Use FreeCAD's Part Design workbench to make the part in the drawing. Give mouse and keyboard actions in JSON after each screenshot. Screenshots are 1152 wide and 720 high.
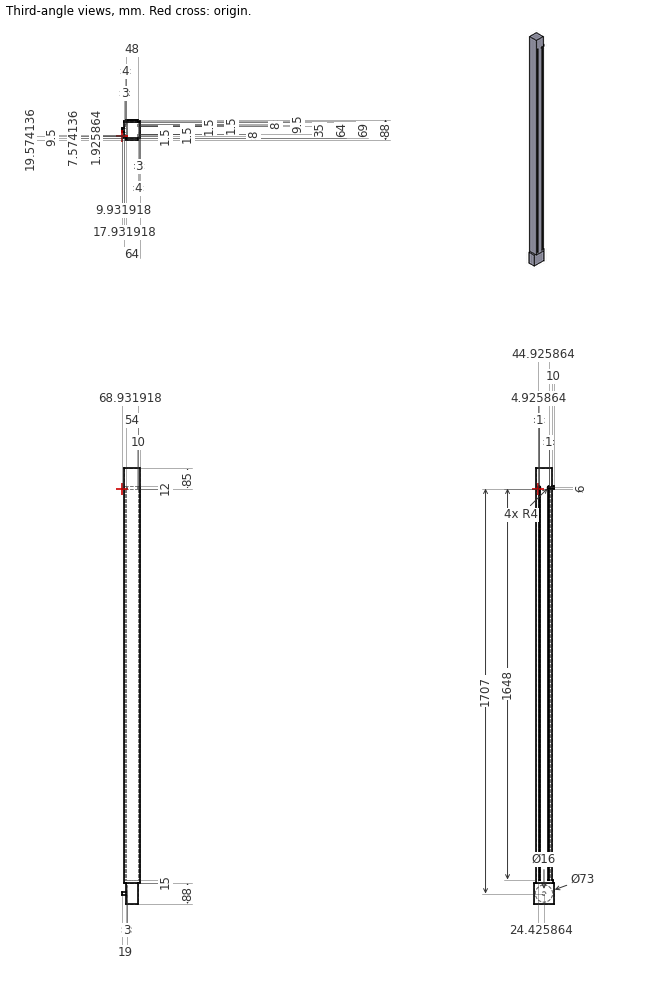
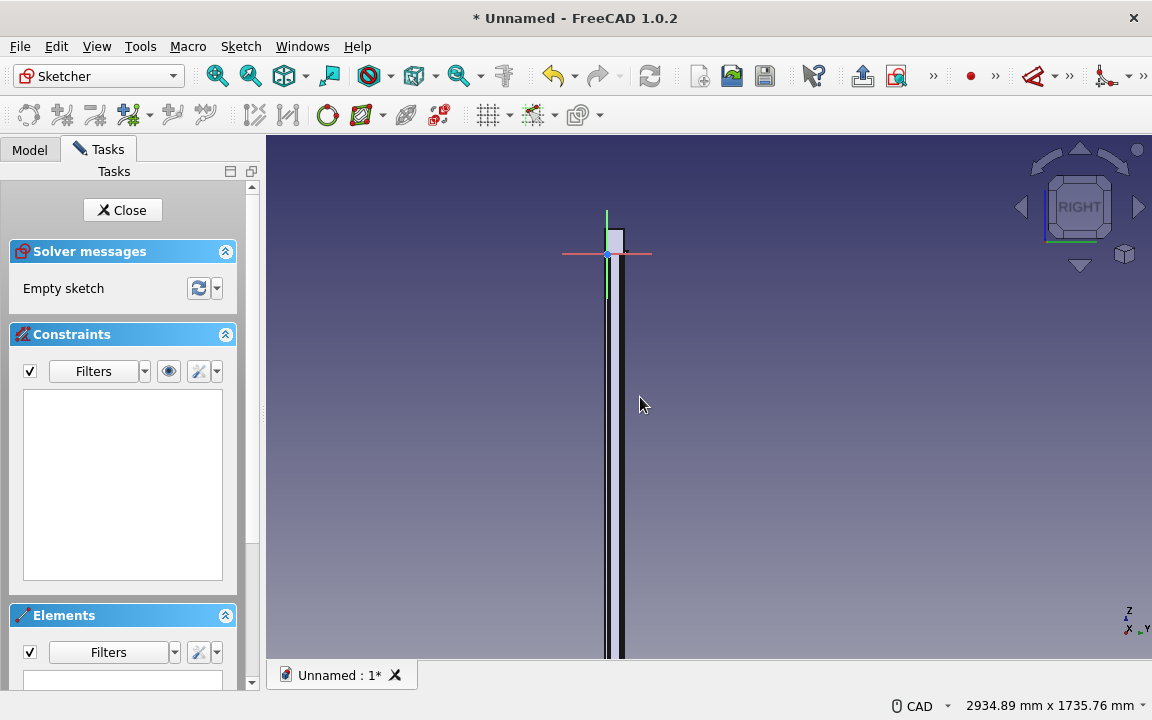
{"action": "scroll", "coordinate": [613, 245], "scroll_direction": "up", "scroll_amount": 15}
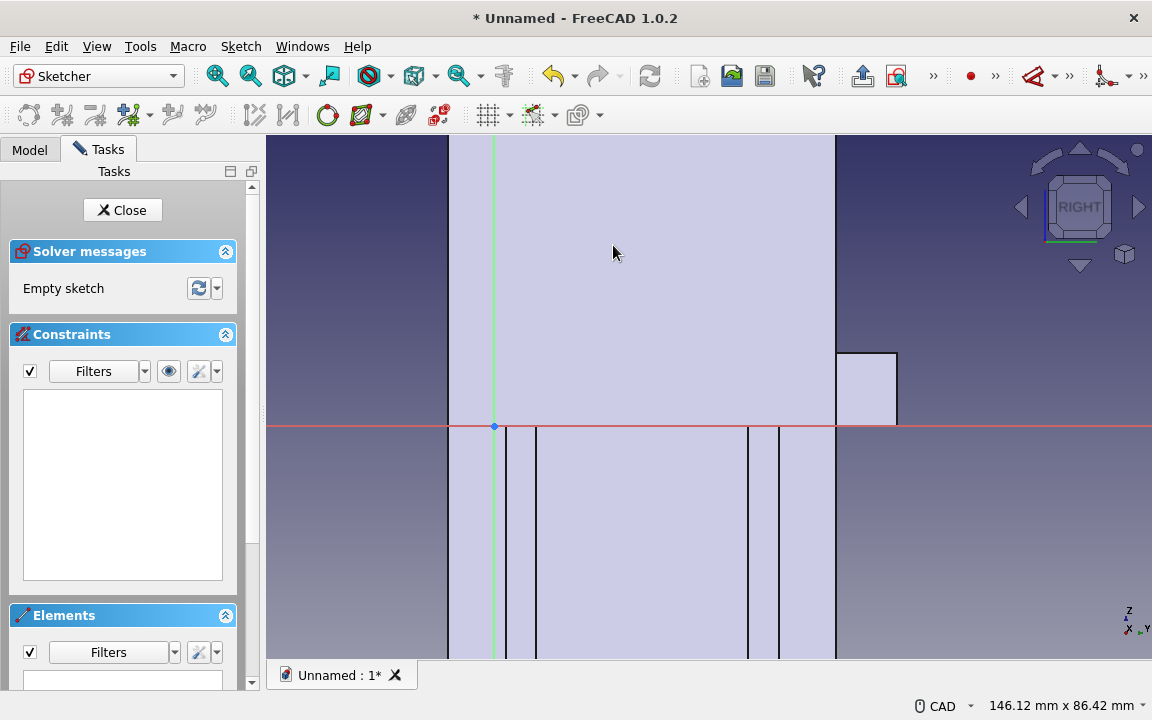
{"action": "scroll", "coordinate": [645, 393], "scroll_direction": "up", "scroll_amount": 2}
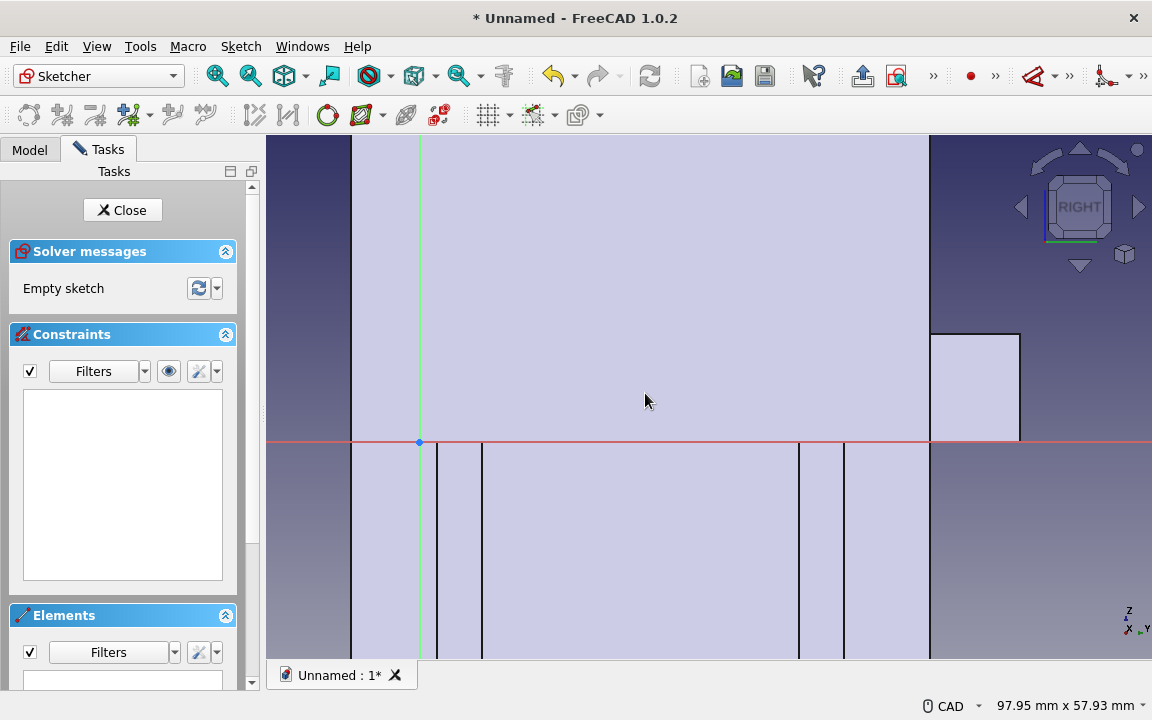
{"action": "key", "text": "g l"}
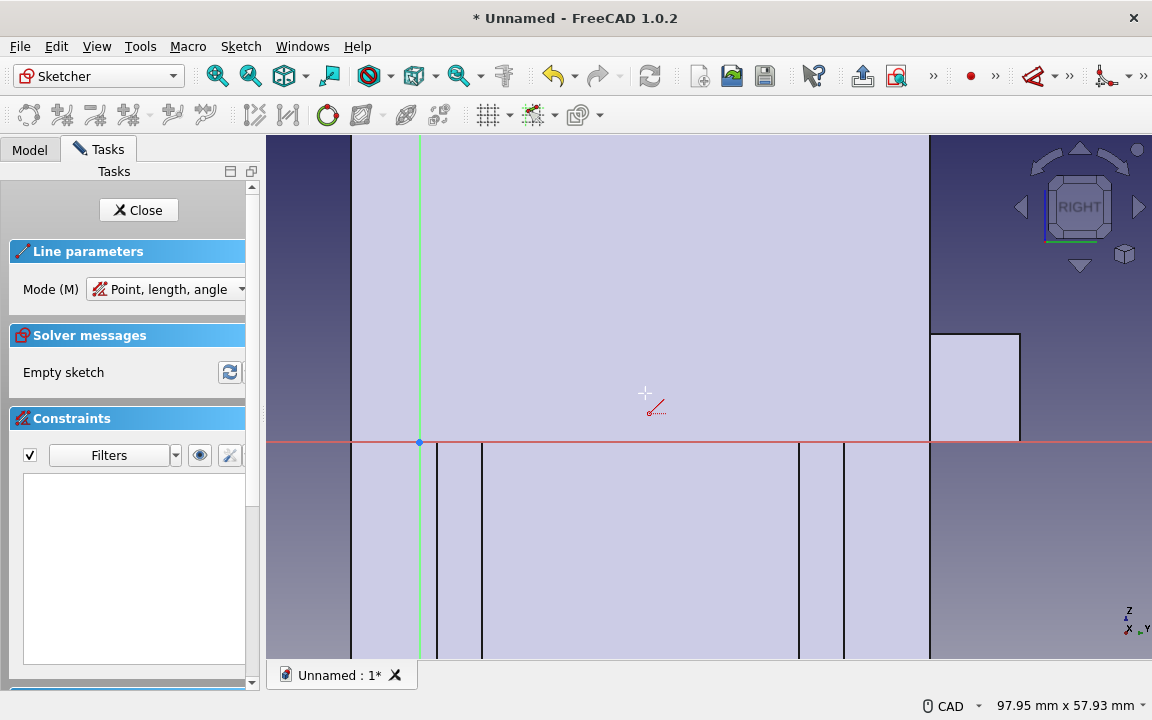
{"action": "left_click", "coordinate": [826, 352]}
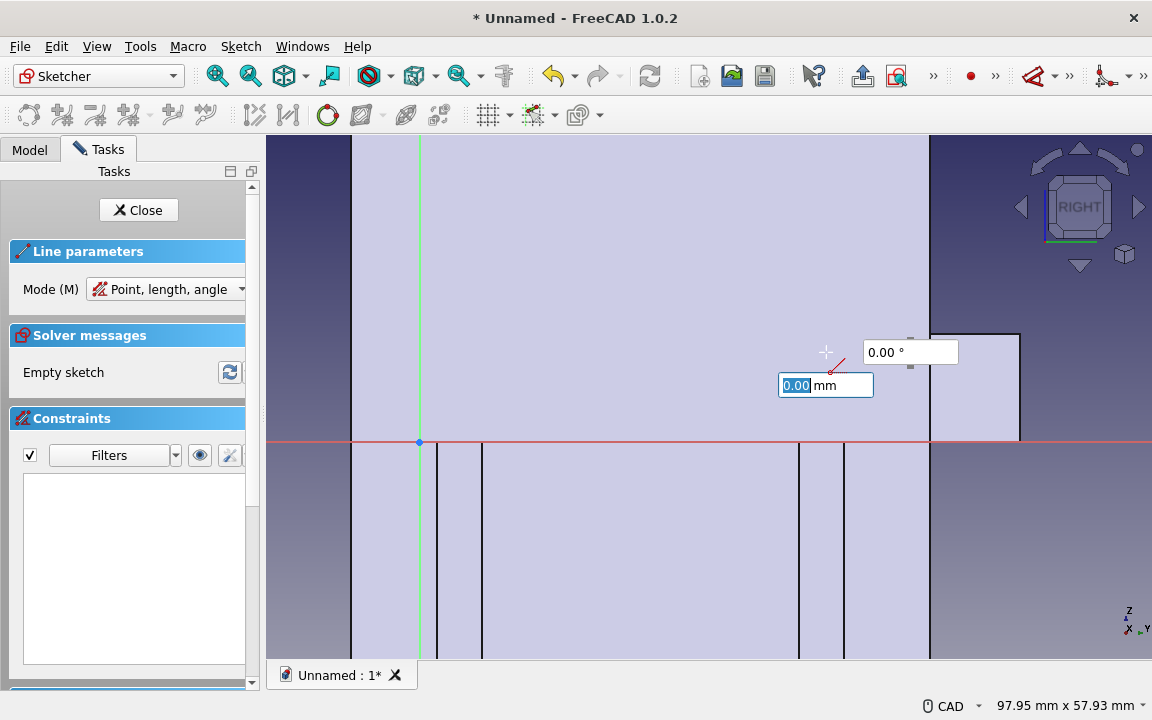
{"action": "scroll", "coordinate": [817, 352], "scroll_direction": "up", "scroll_amount": 3}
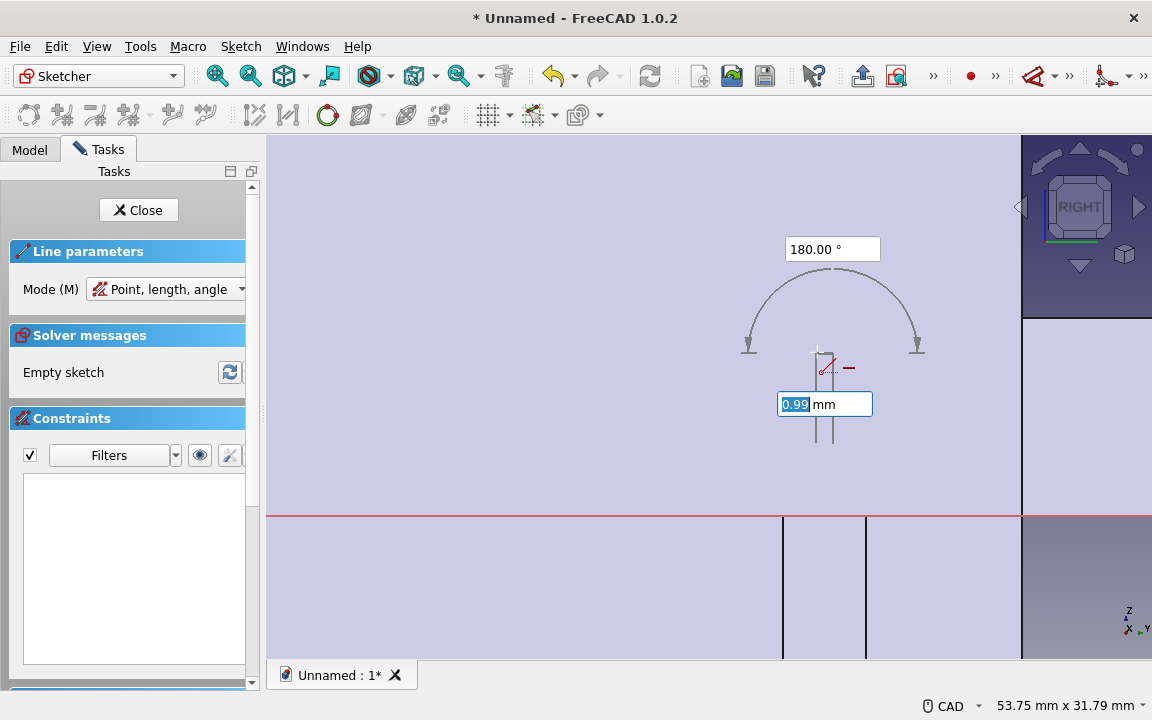
{"action": "left_click", "coordinate": [816, 352]}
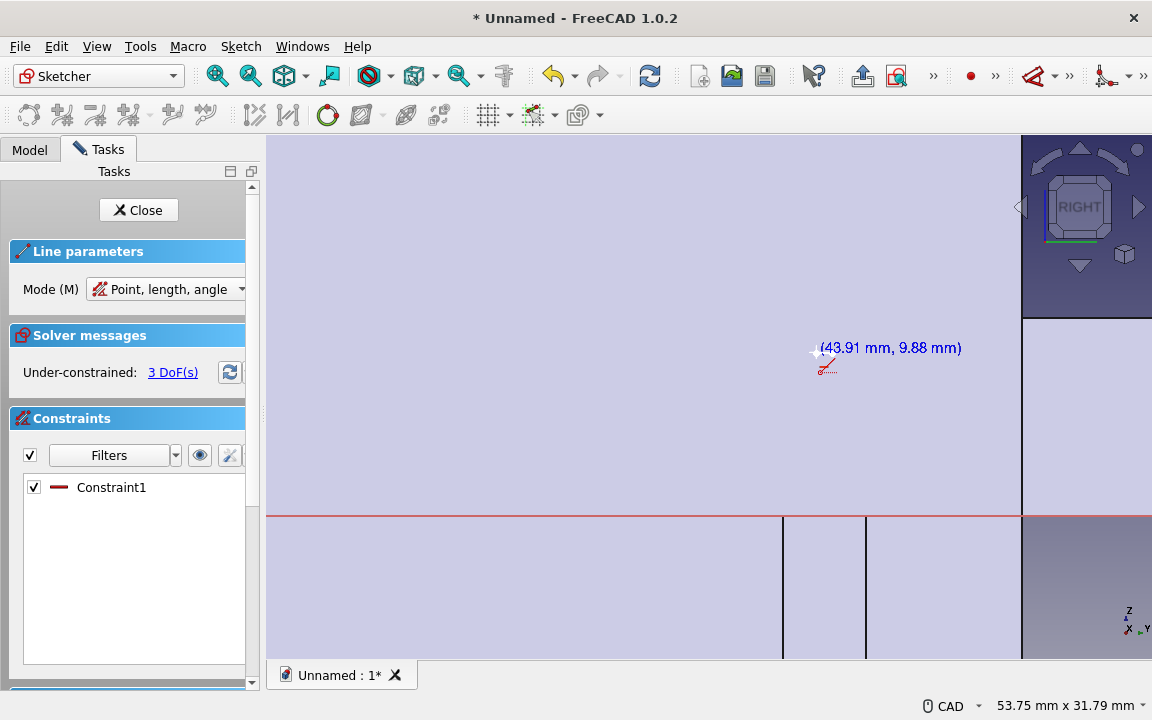
{"action": "key", "text": "g m"}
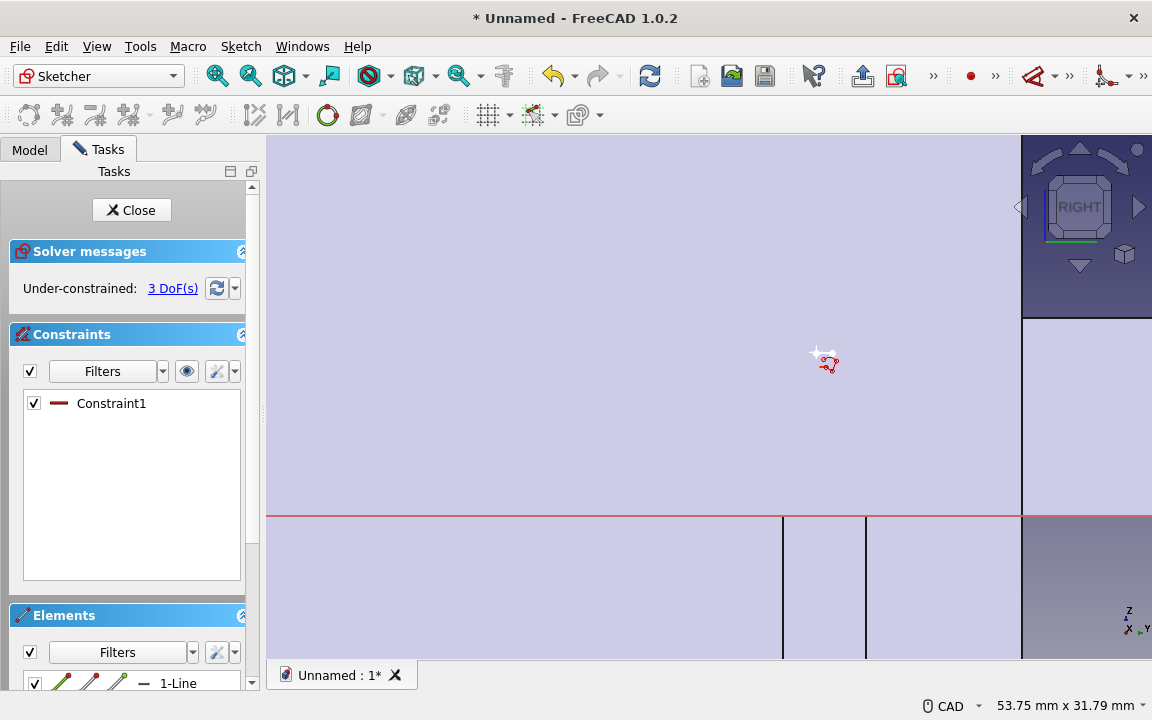
{"action": "left_click", "coordinate": [750, 417]}
{"action": "left_click", "coordinate": [750, 516]}
{"action": "left_click", "coordinate": [899, 507]}
{"action": "left_click", "coordinate": [899, 417]}
{"action": "right_click", "coordinate": [899, 417]}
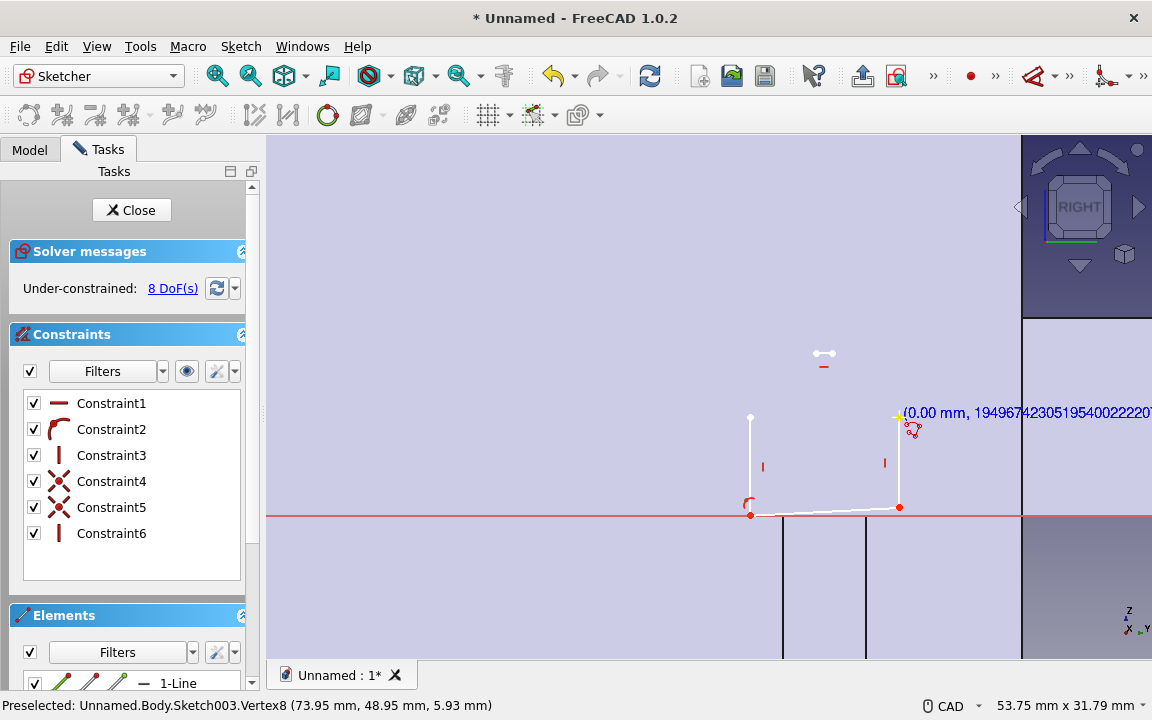
{"action": "key", "text": "g 3 a"}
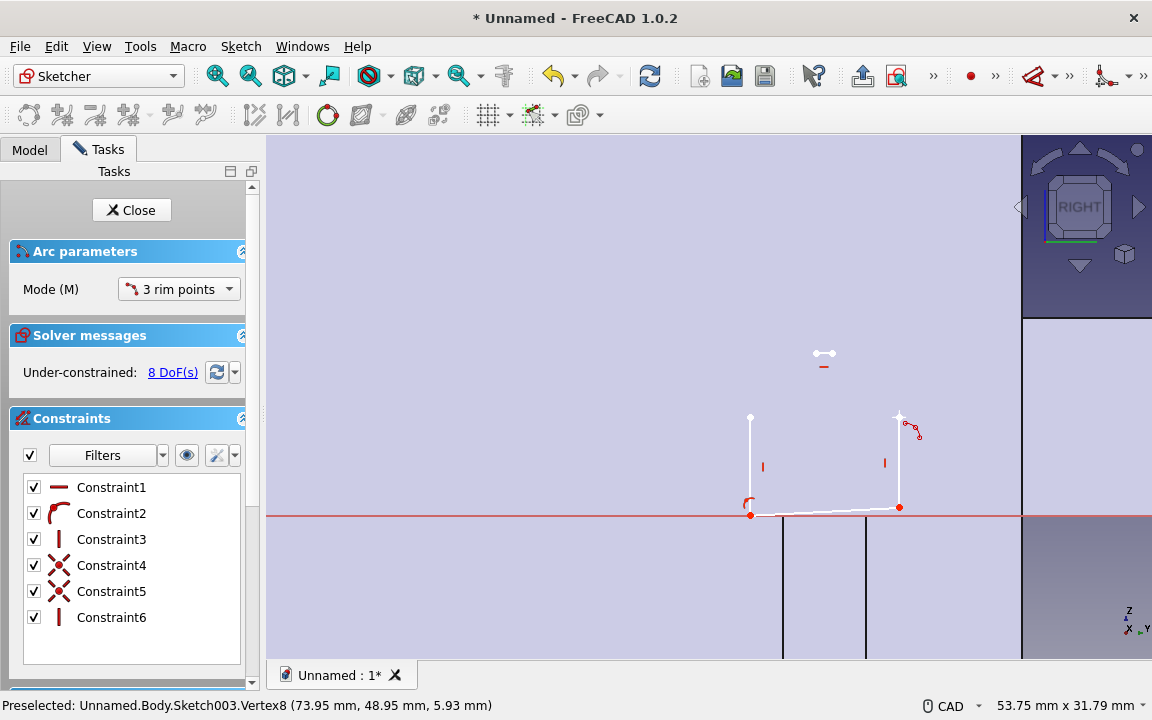
{"action": "scroll", "coordinate": [816, 351], "scroll_direction": "up", "scroll_amount": 4}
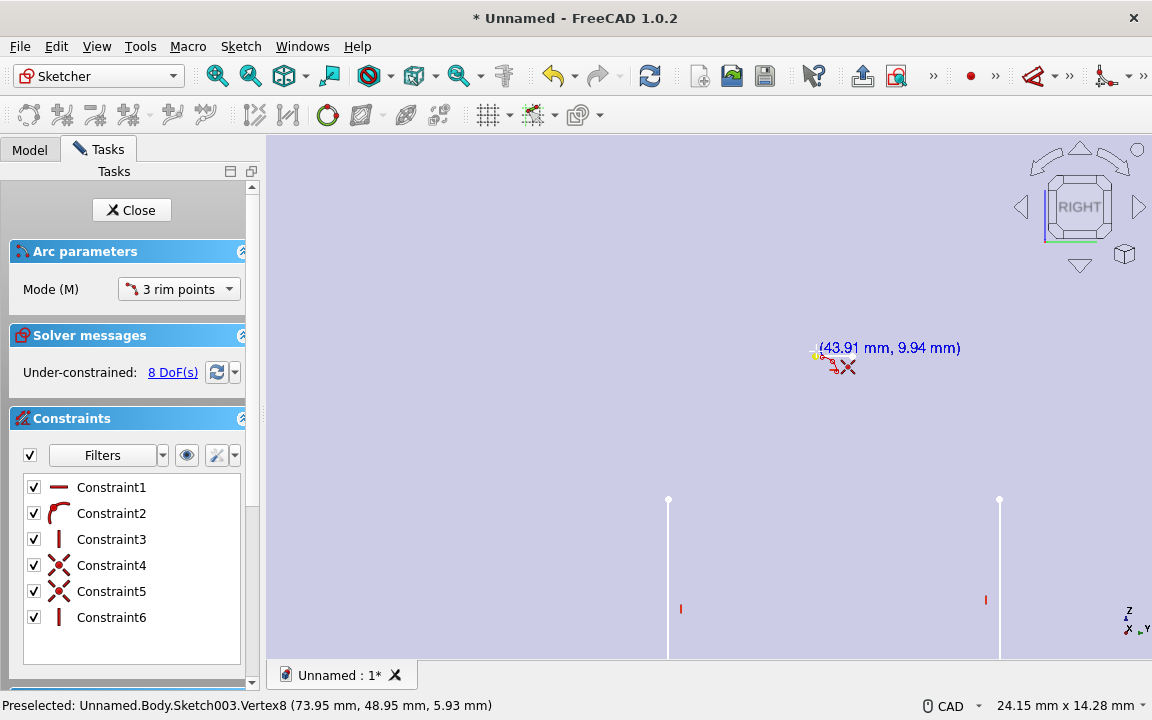
{"action": "left_click", "coordinate": [815, 356]}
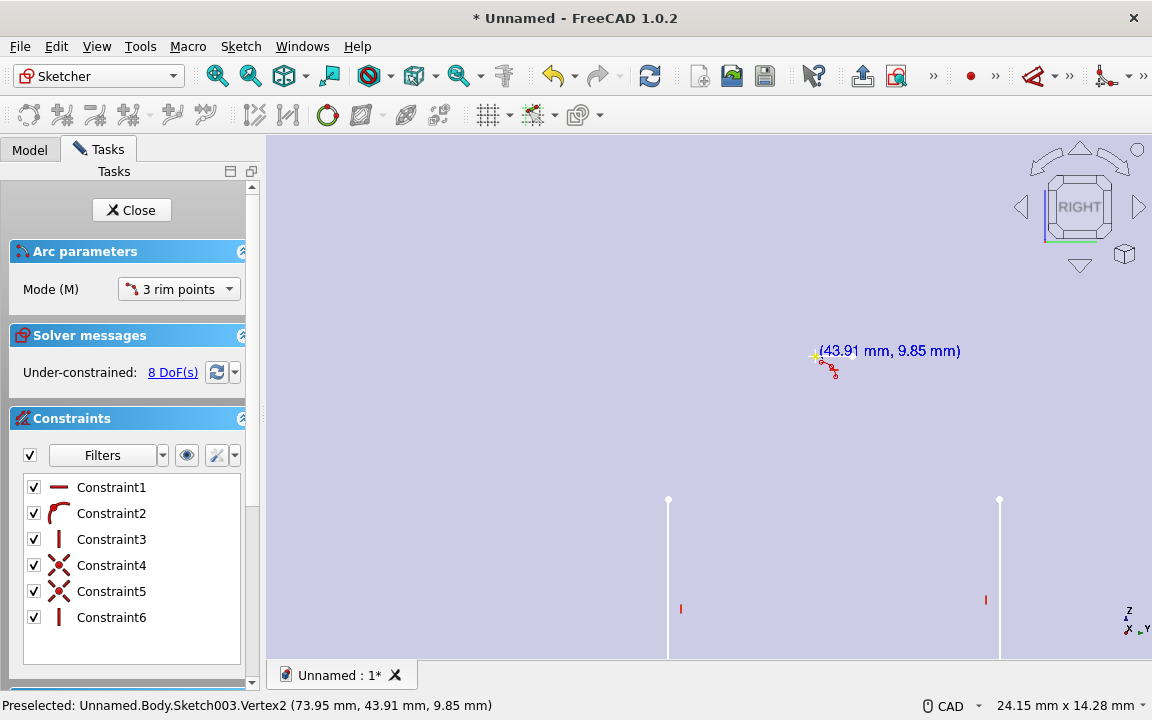
{"action": "scroll", "coordinate": [817, 352], "scroll_direction": "down", "scroll_amount": 7}